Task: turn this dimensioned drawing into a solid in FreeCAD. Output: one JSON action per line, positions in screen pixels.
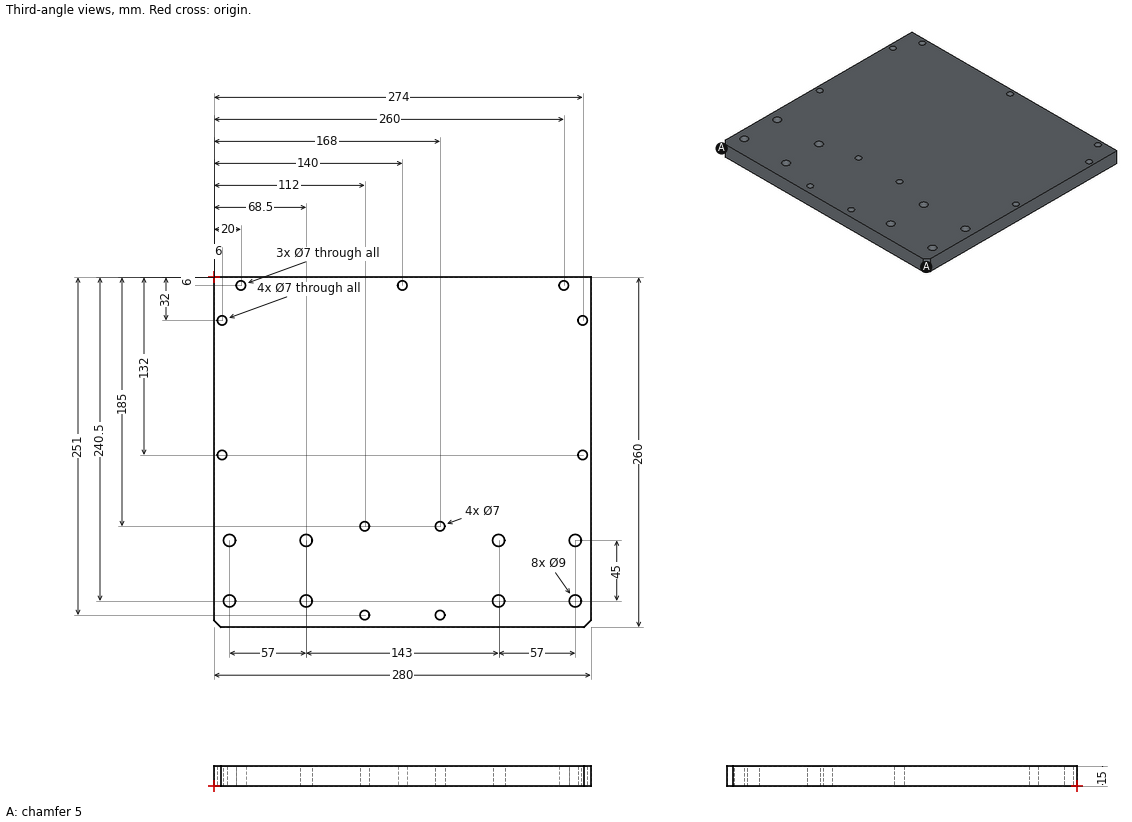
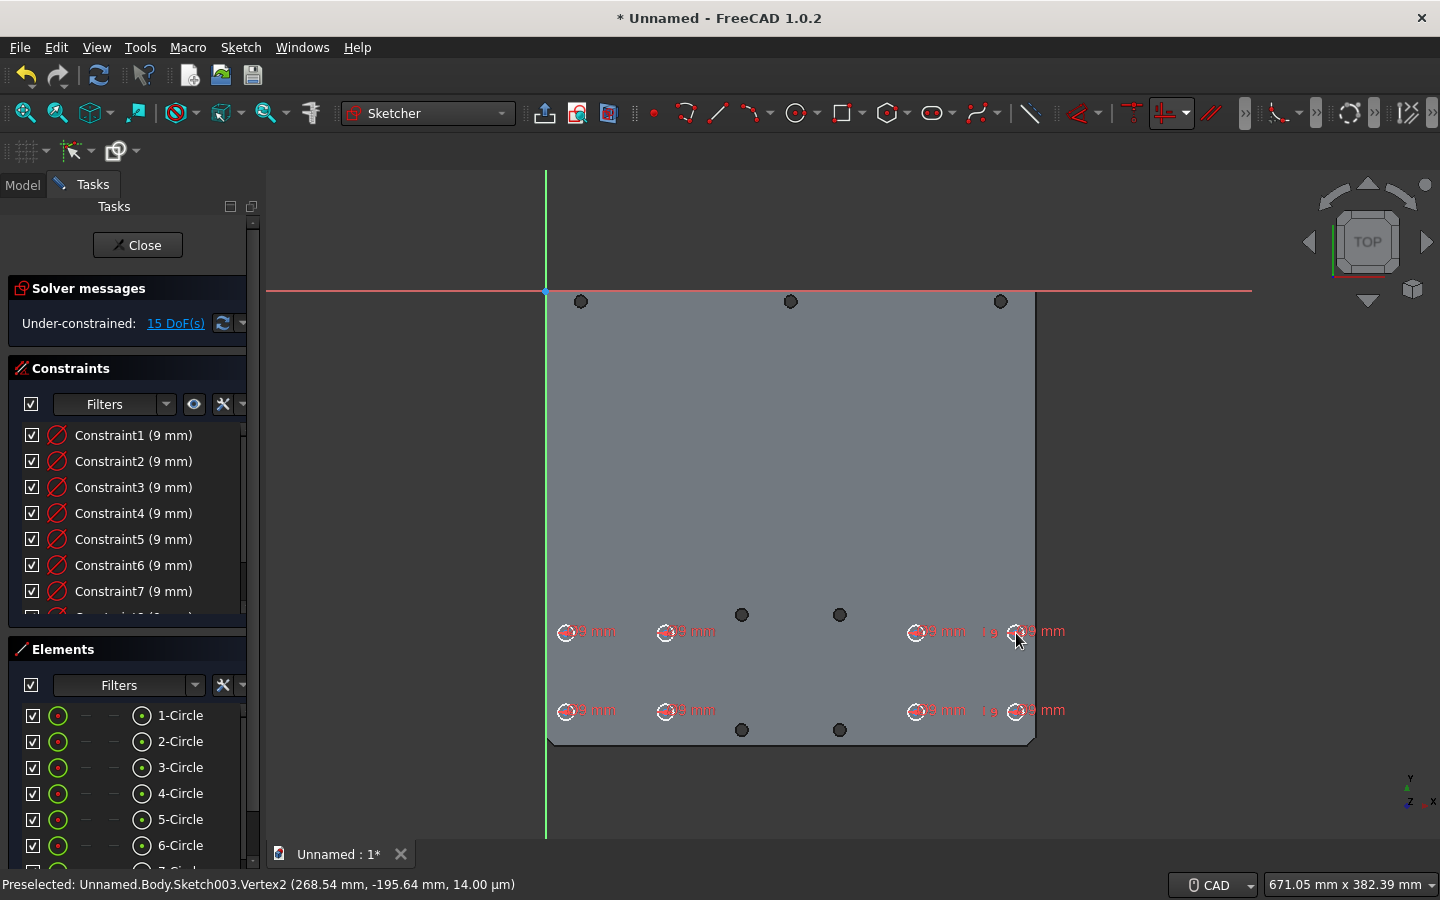
{"action": "left_click", "coordinate": [1016, 633]}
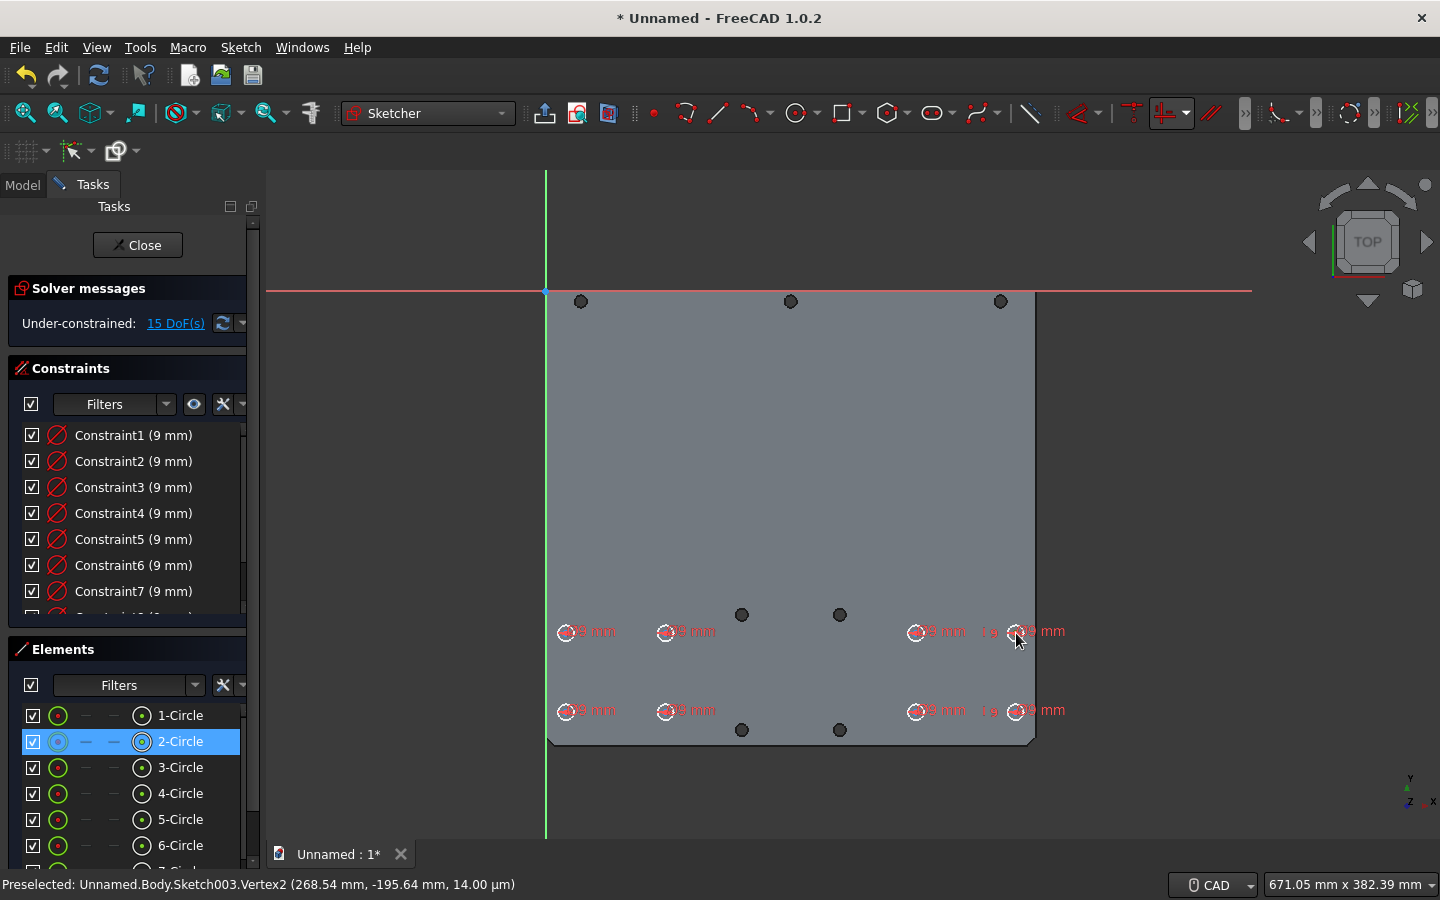
{"action": "left_click", "coordinate": [916, 633]}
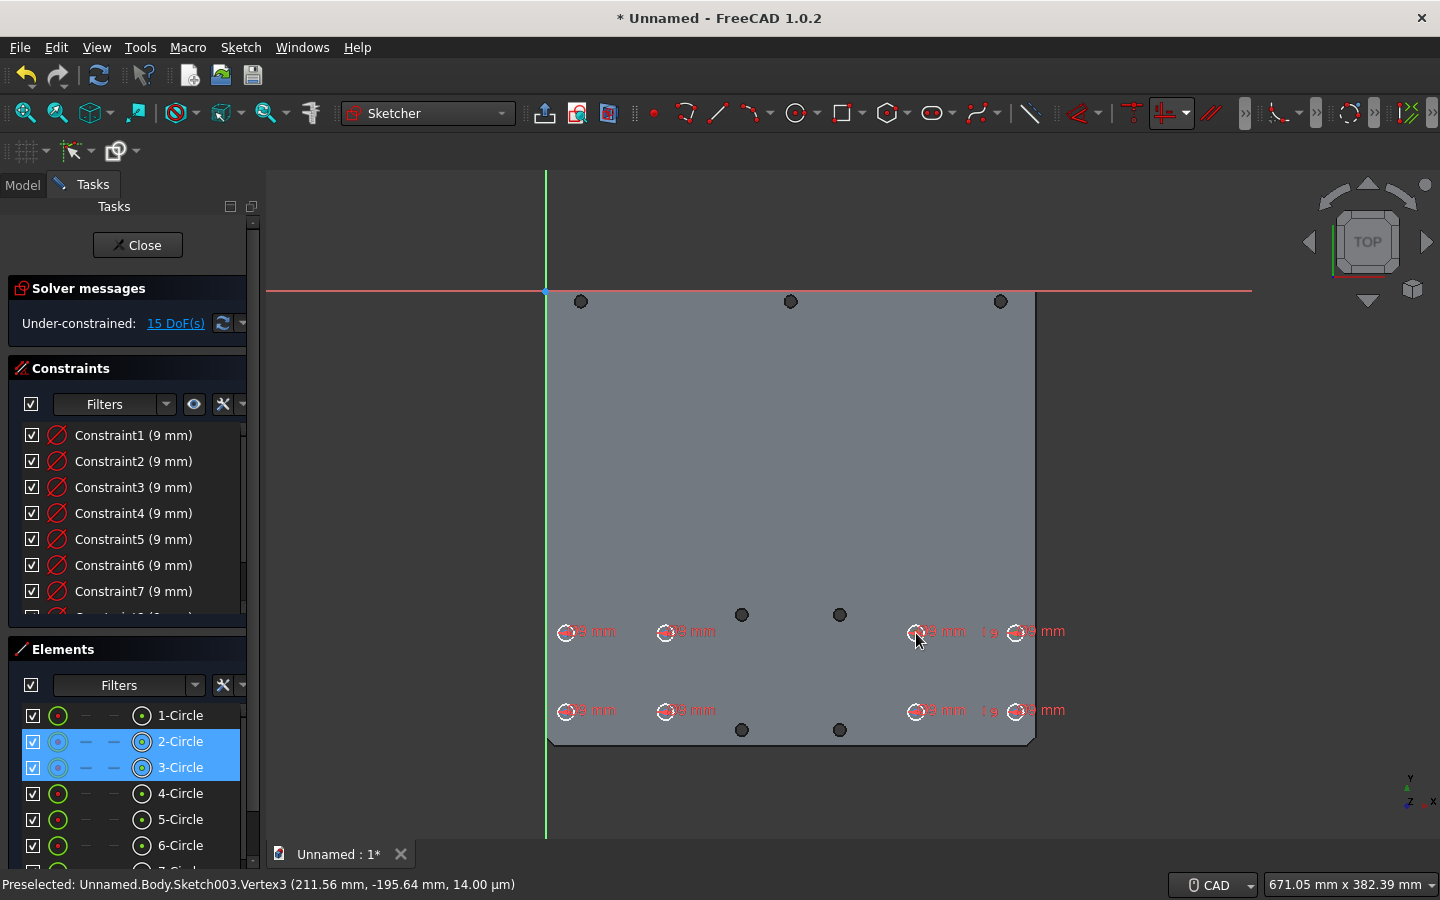
{"action": "key", "text": "h"}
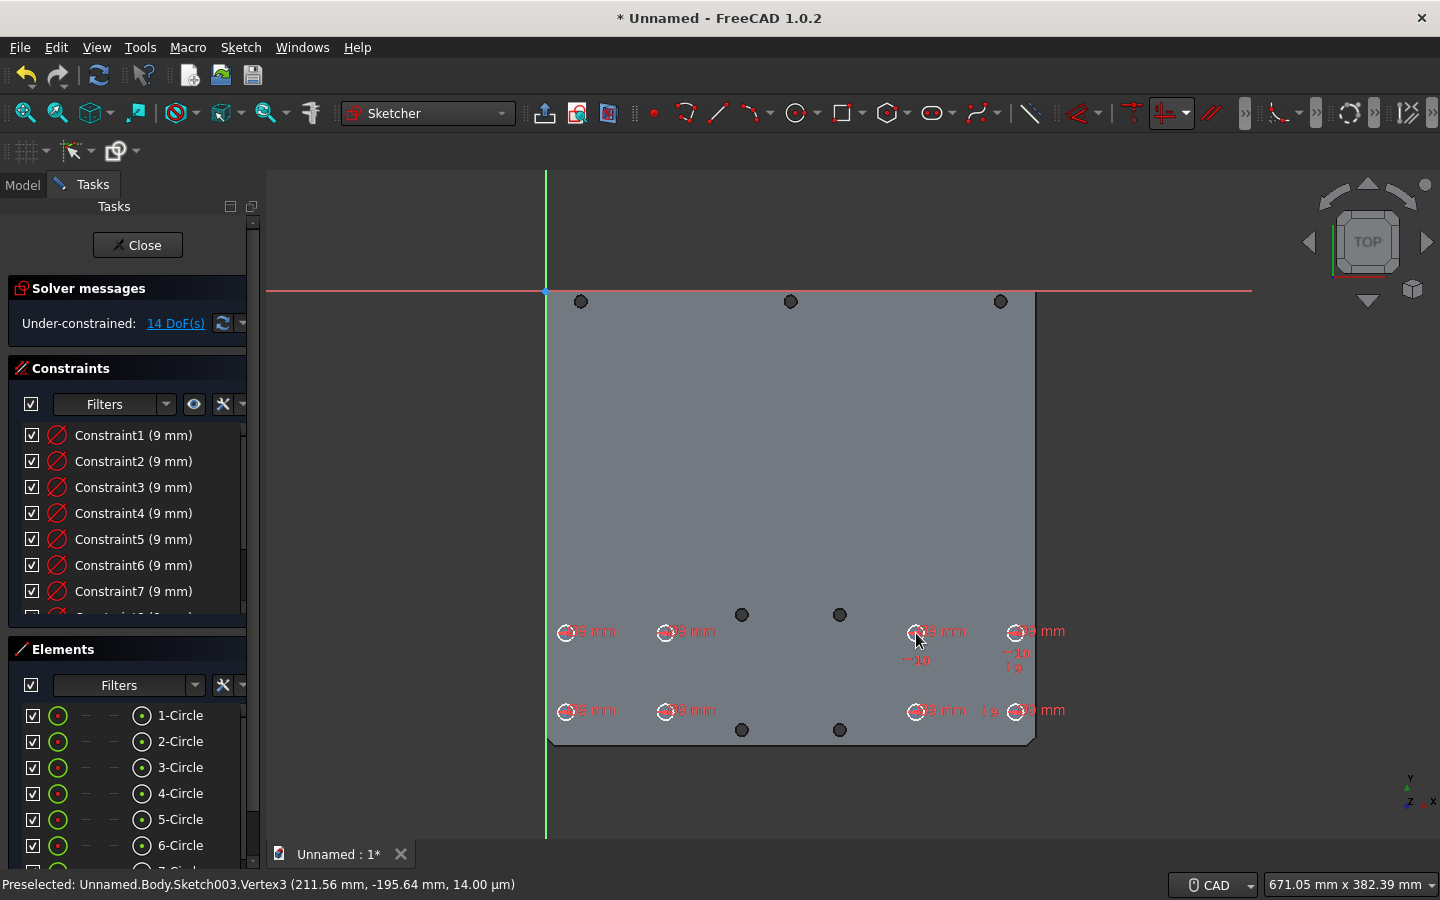
{"action": "left_click", "coordinate": [916, 633]}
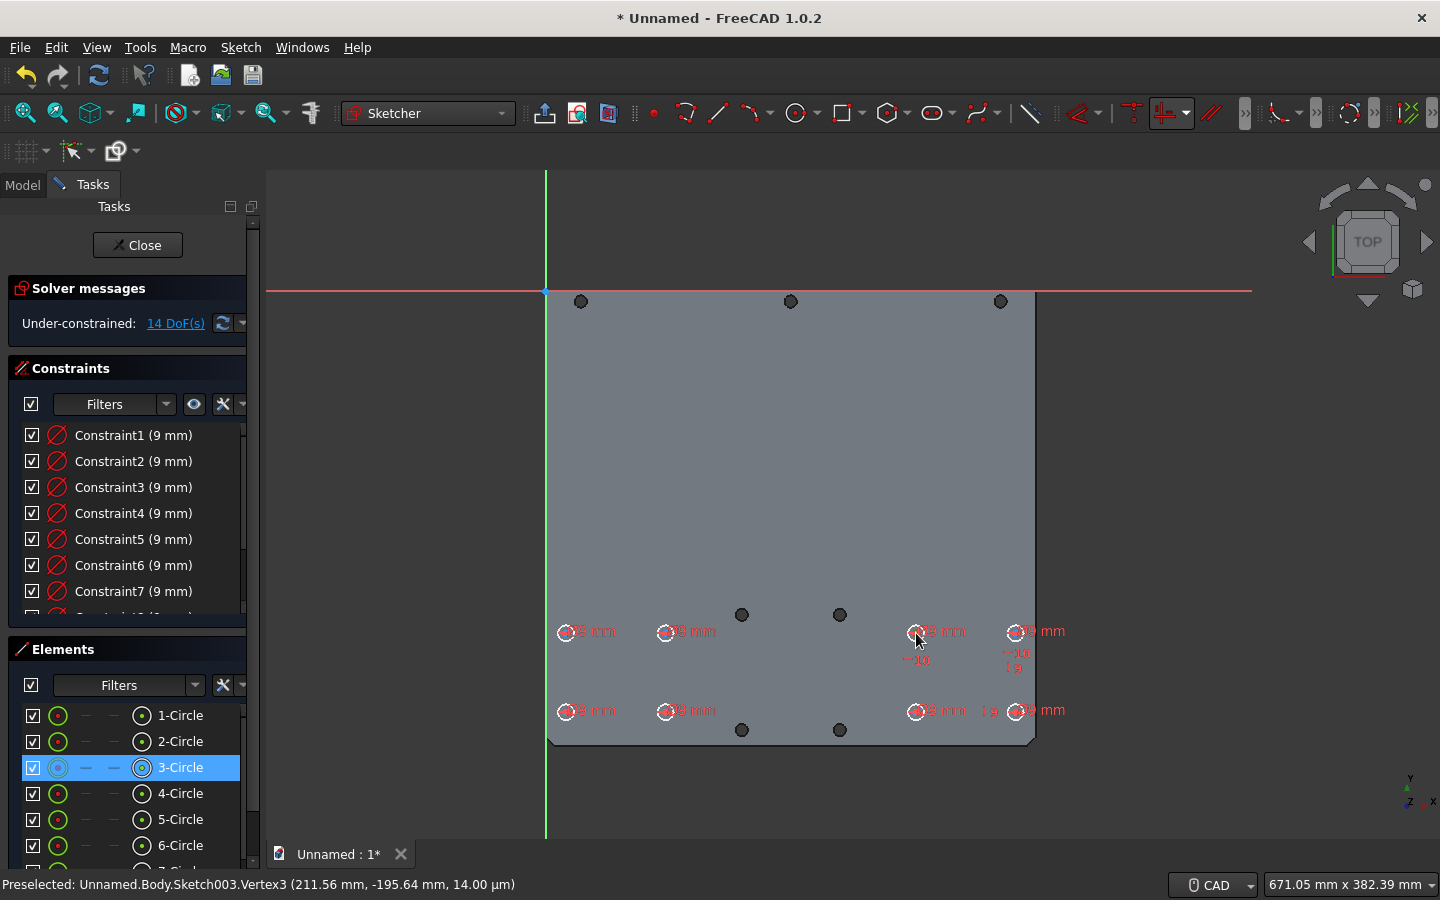
{"action": "left_click", "coordinate": [916, 712]}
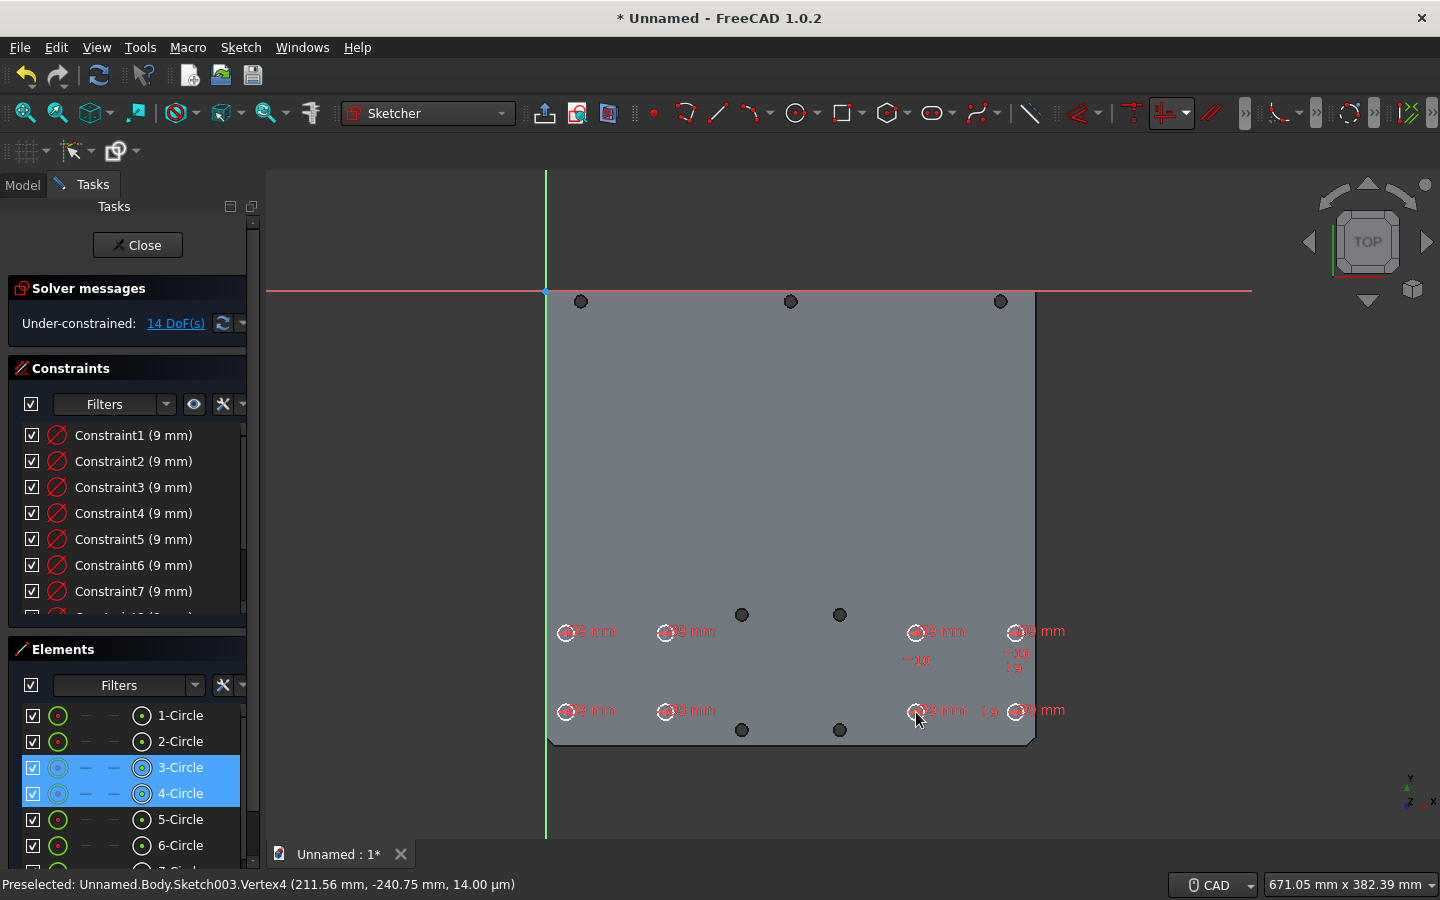
{"action": "key", "text": "v"}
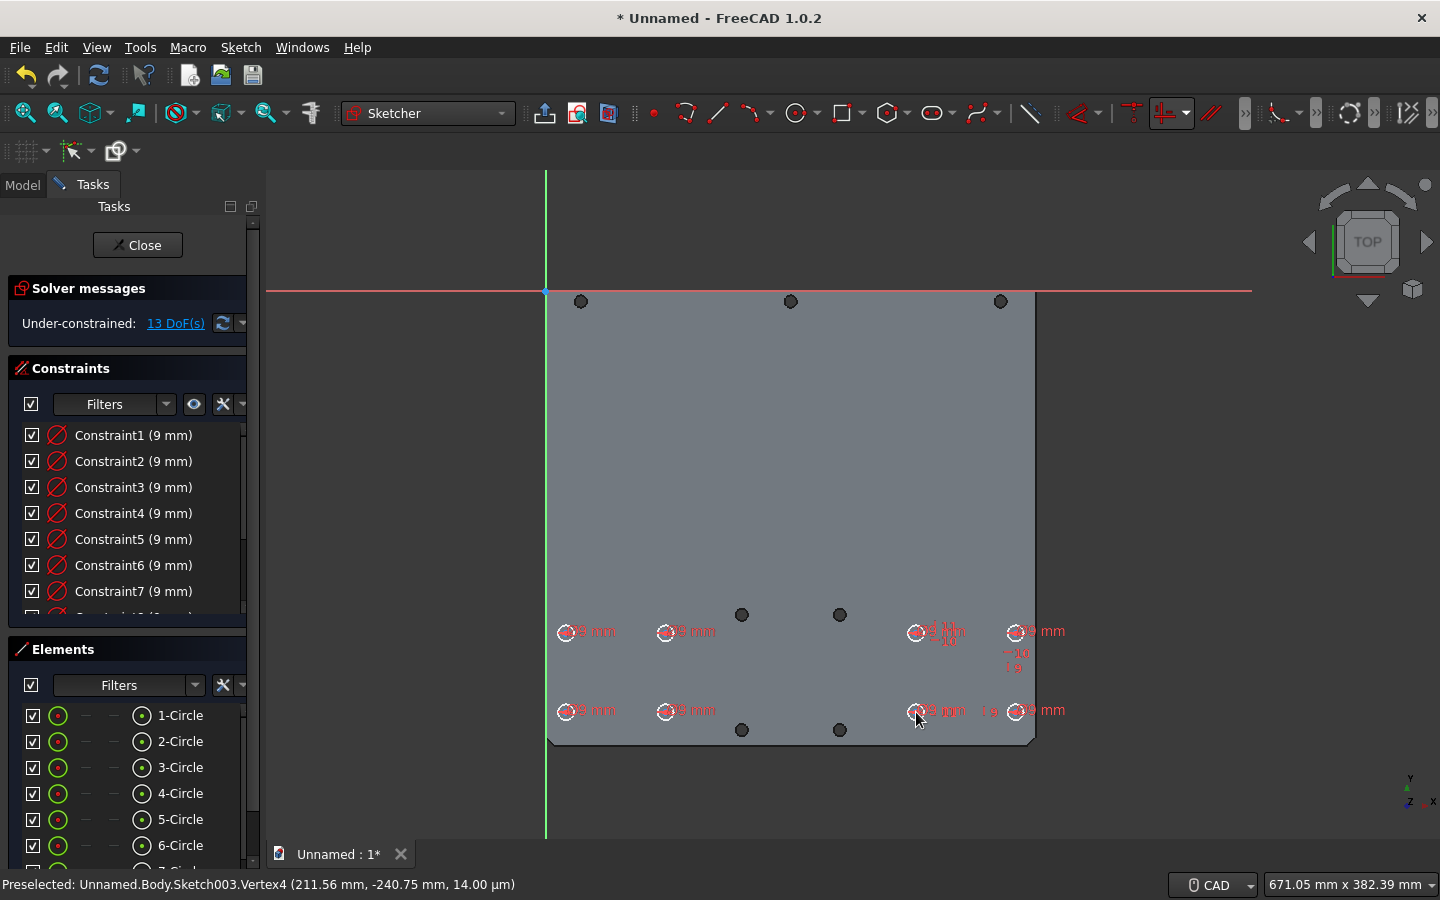
{"action": "left_click", "coordinate": [1016, 712]}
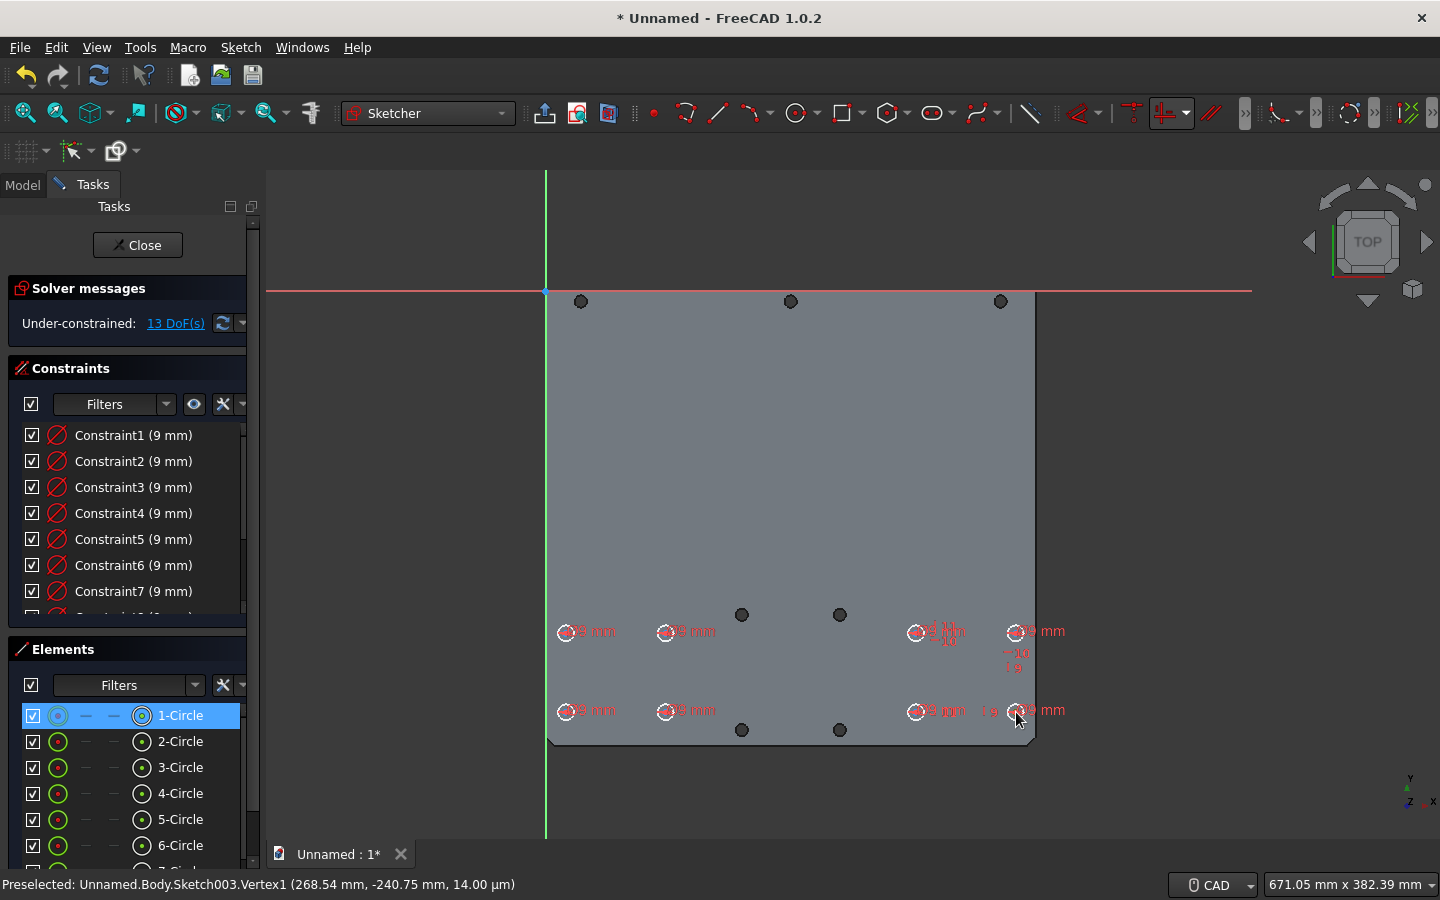
{"action": "left_click", "coordinate": [916, 712]}